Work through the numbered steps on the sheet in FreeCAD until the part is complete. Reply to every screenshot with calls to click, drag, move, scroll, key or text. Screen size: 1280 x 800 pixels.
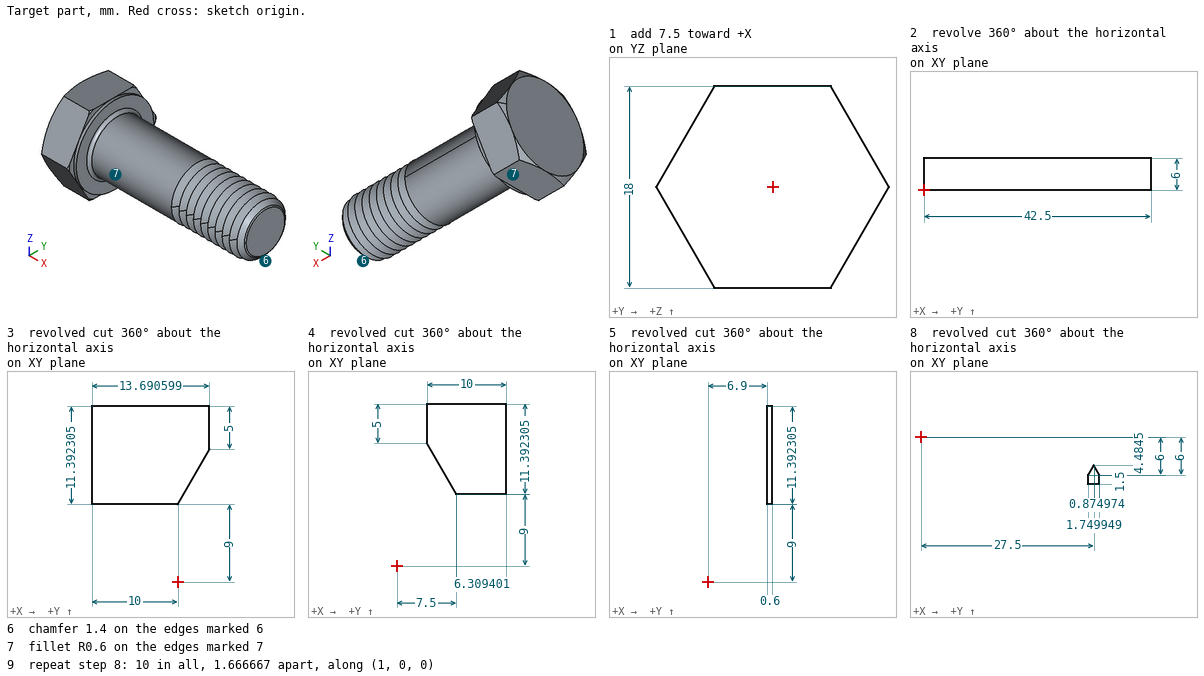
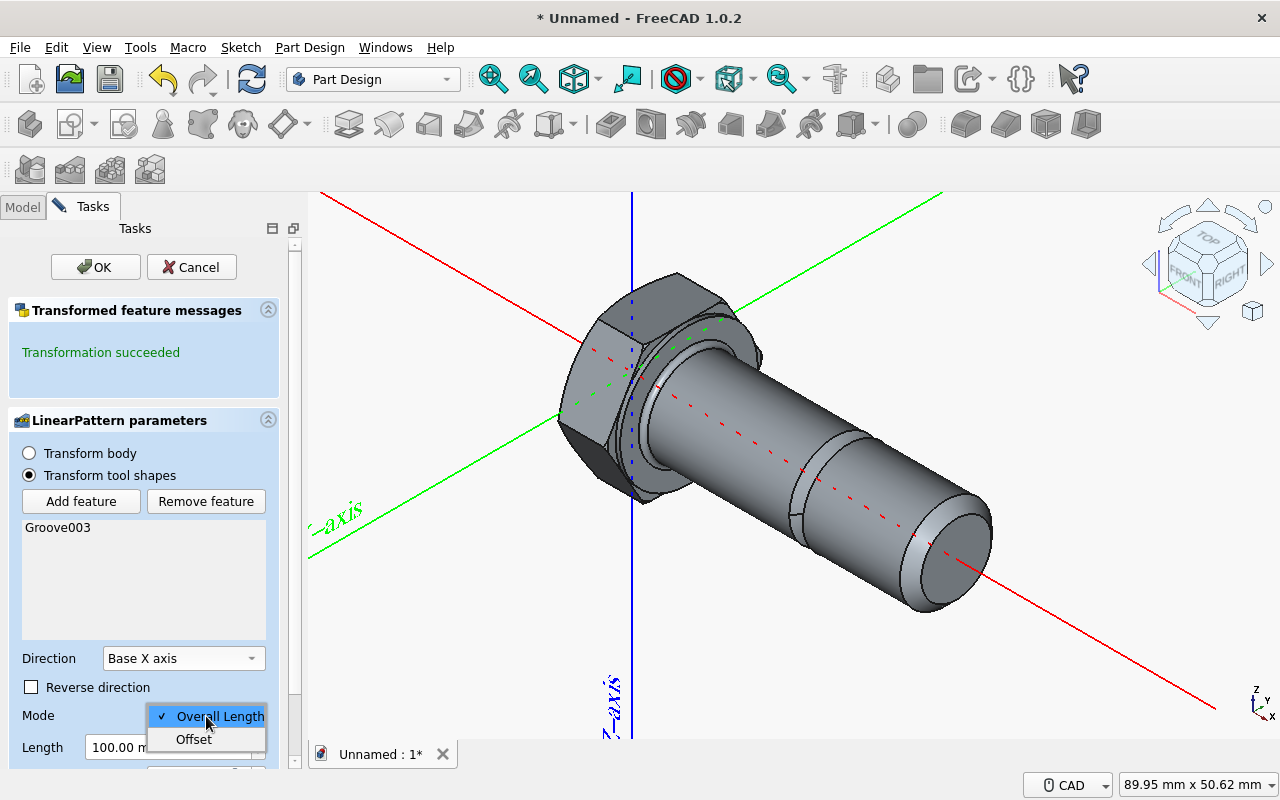
click(206, 740)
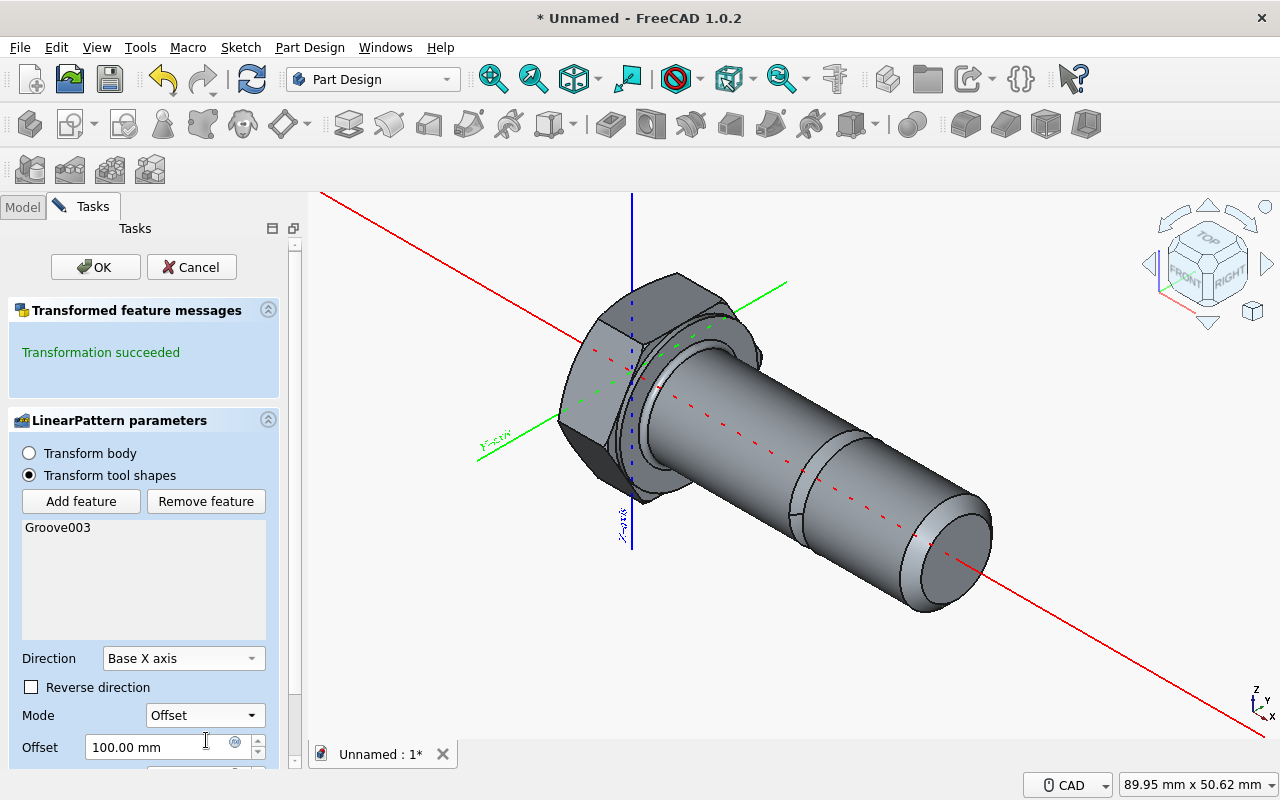
triple_click(168, 747)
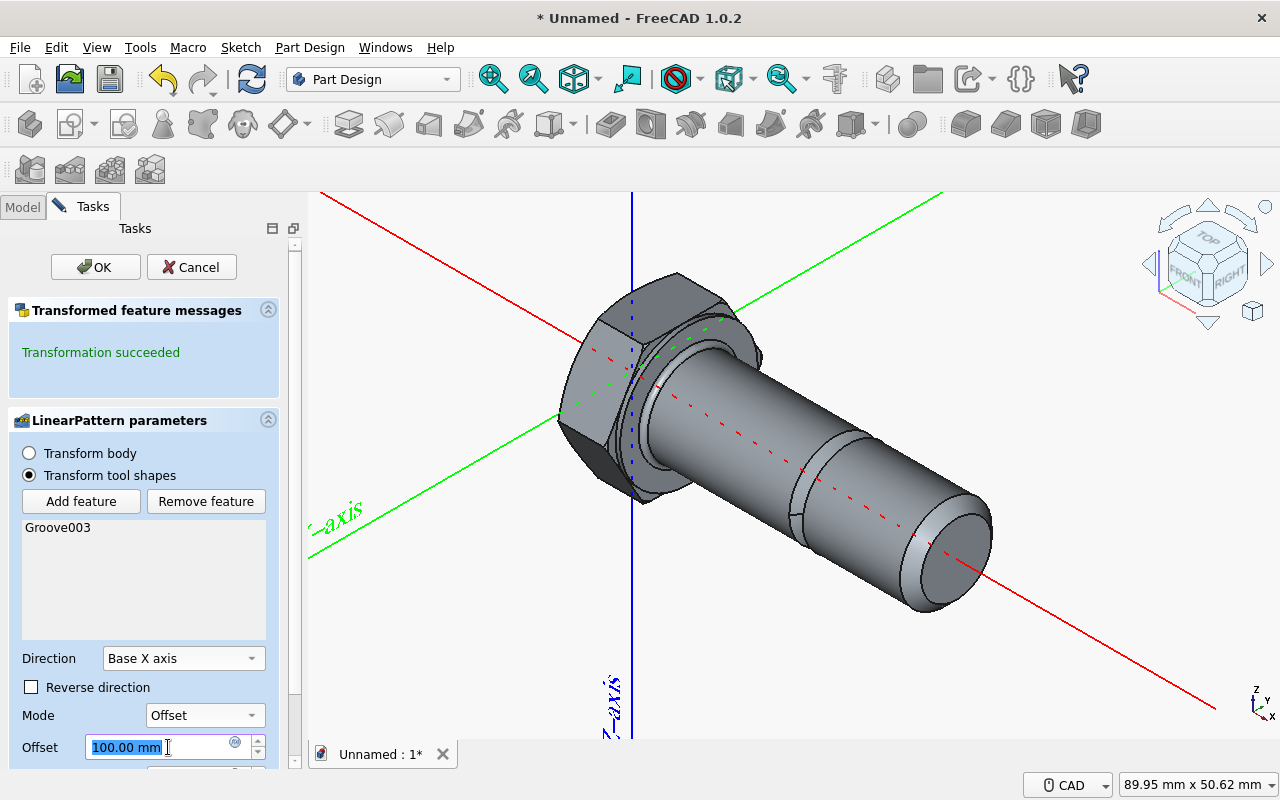
text(1.666667)
key(Tab)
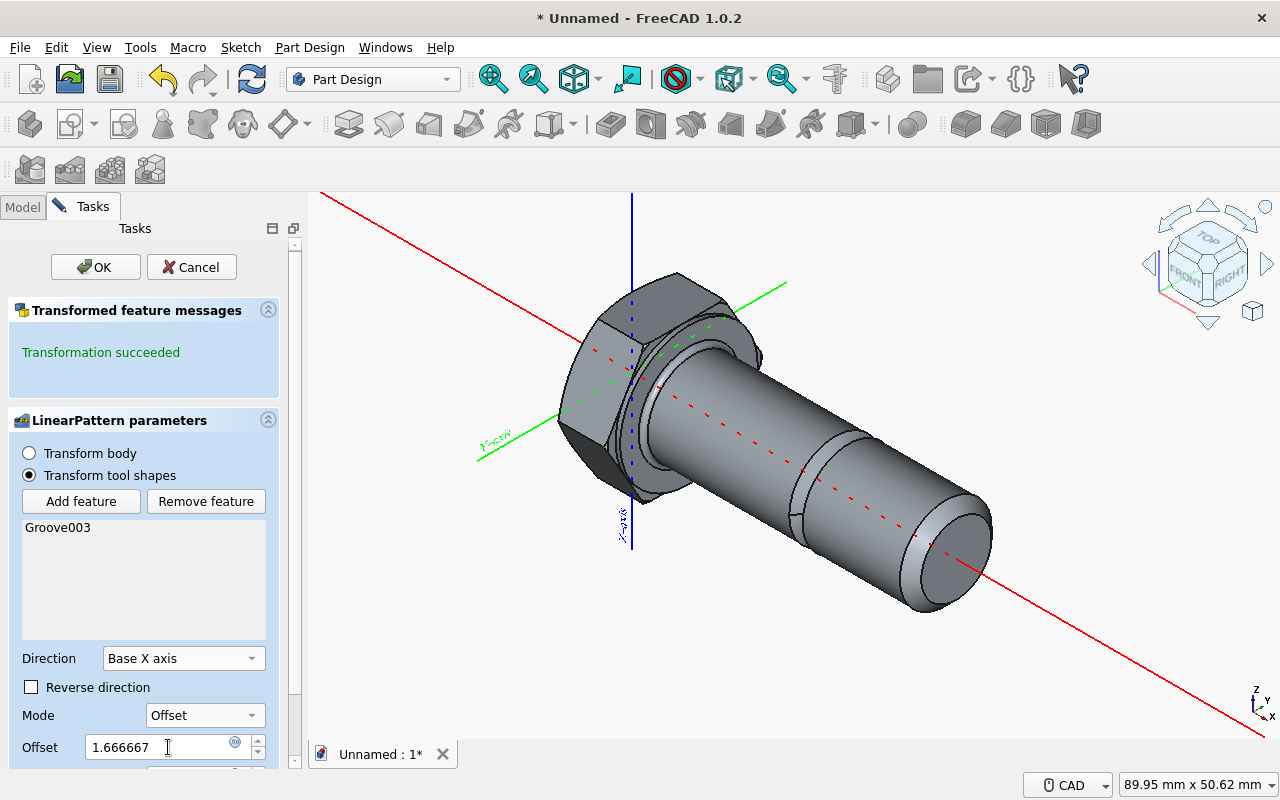
scroll(295, 503, down, 2)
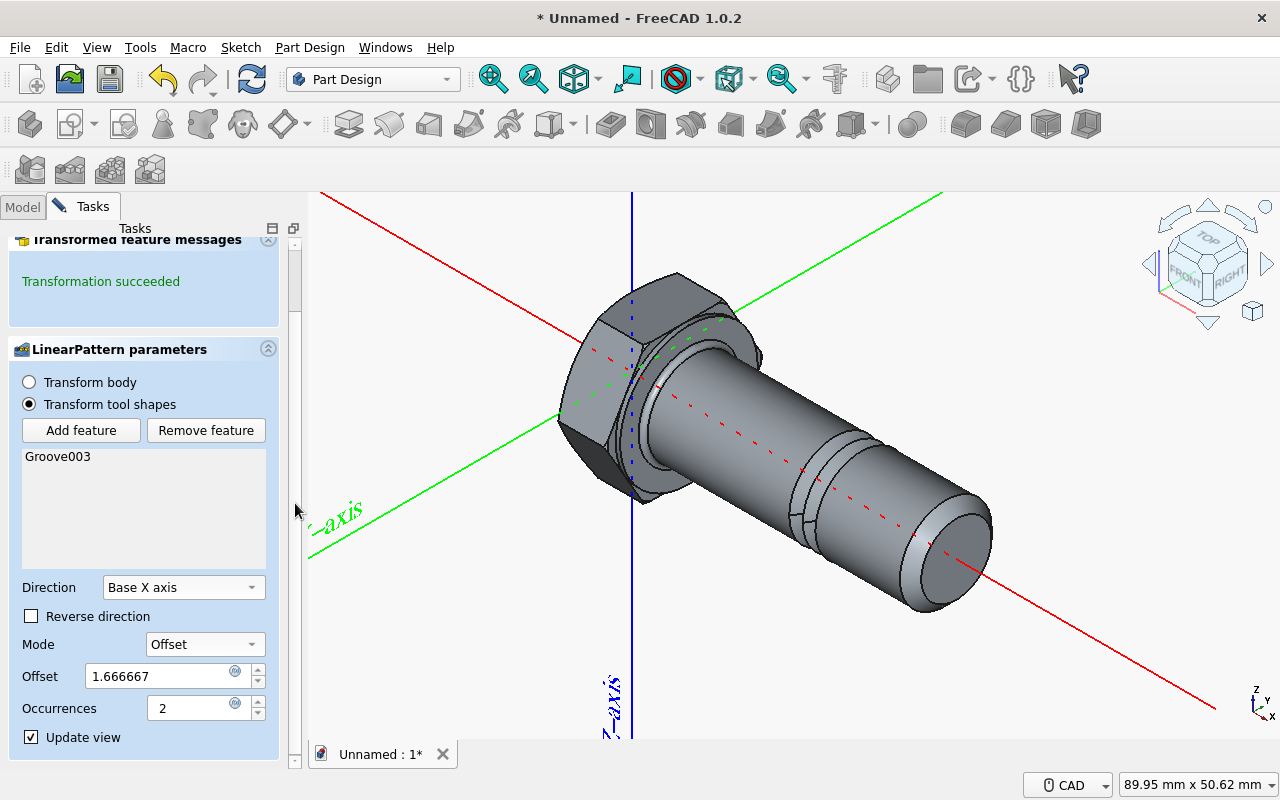
triple_click(198, 708)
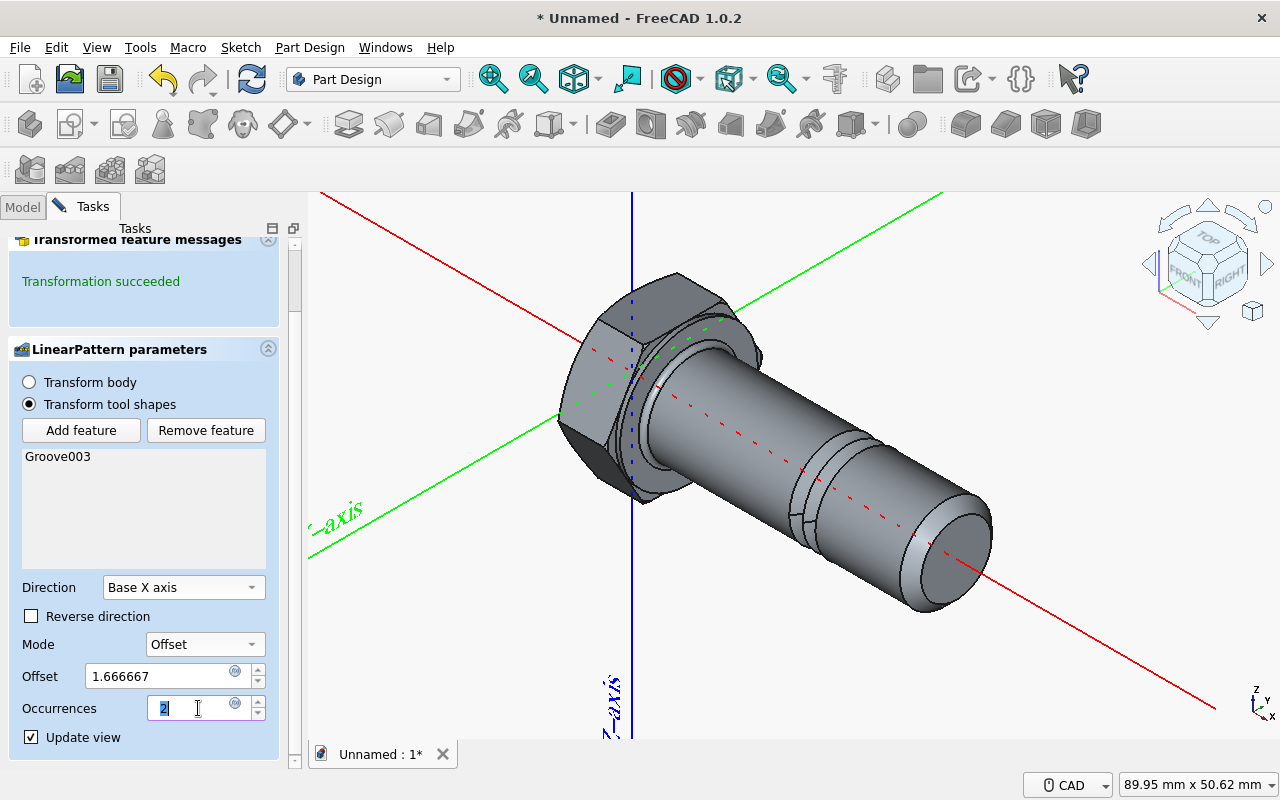
text(10)
key(Tab)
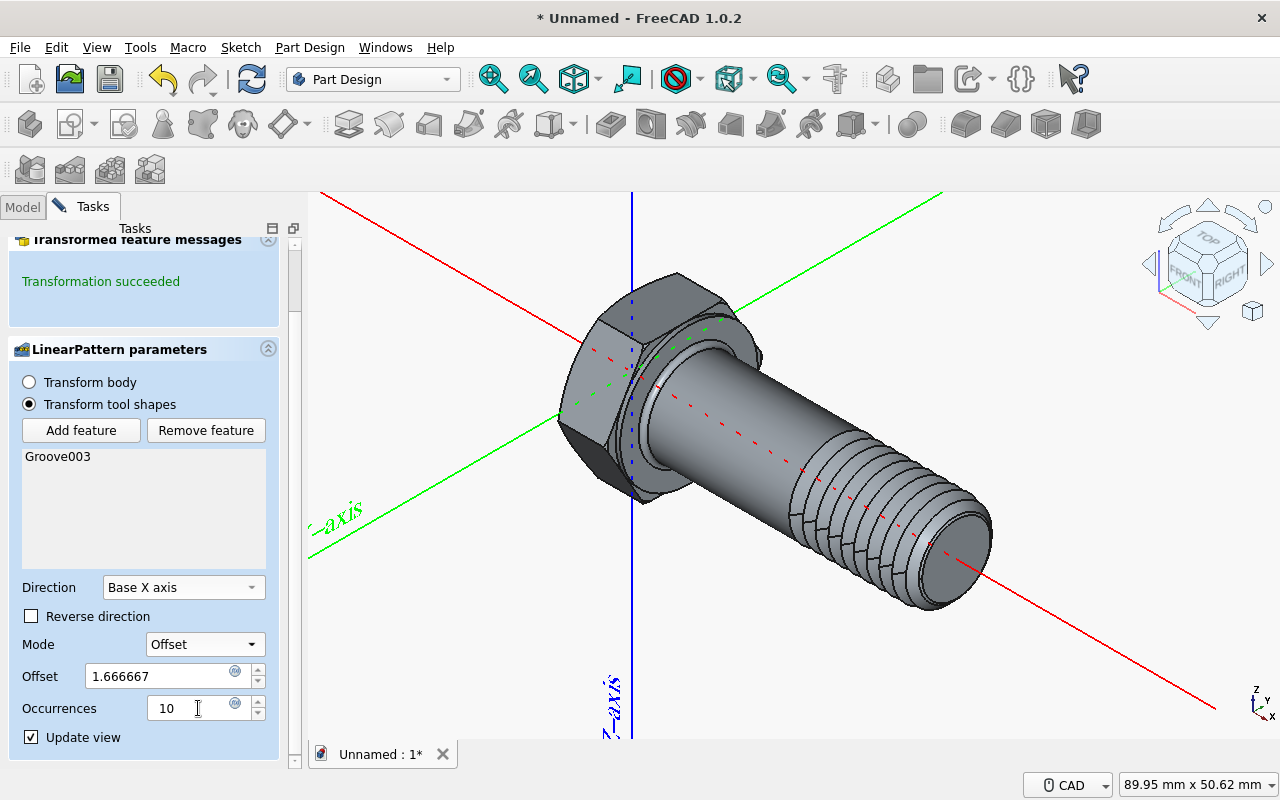
scroll(295, 503, up, 2)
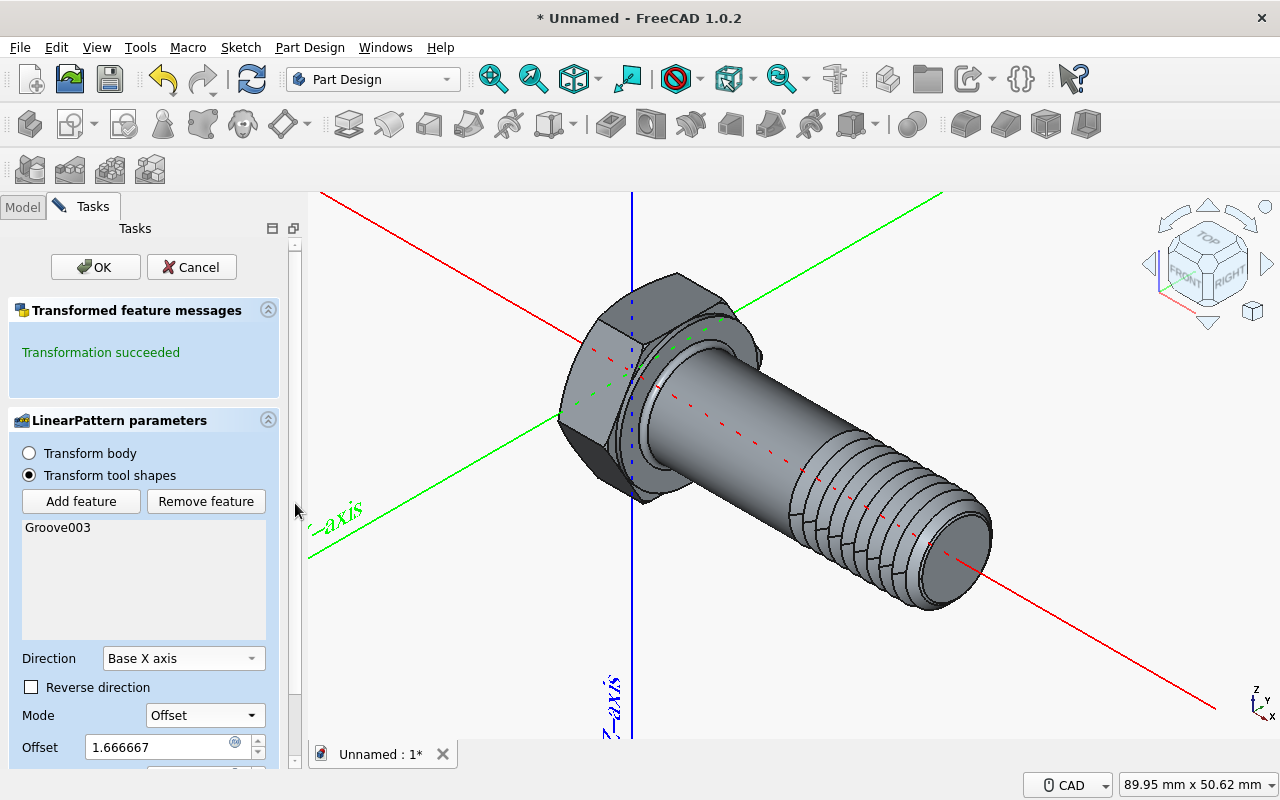
click(96, 267)